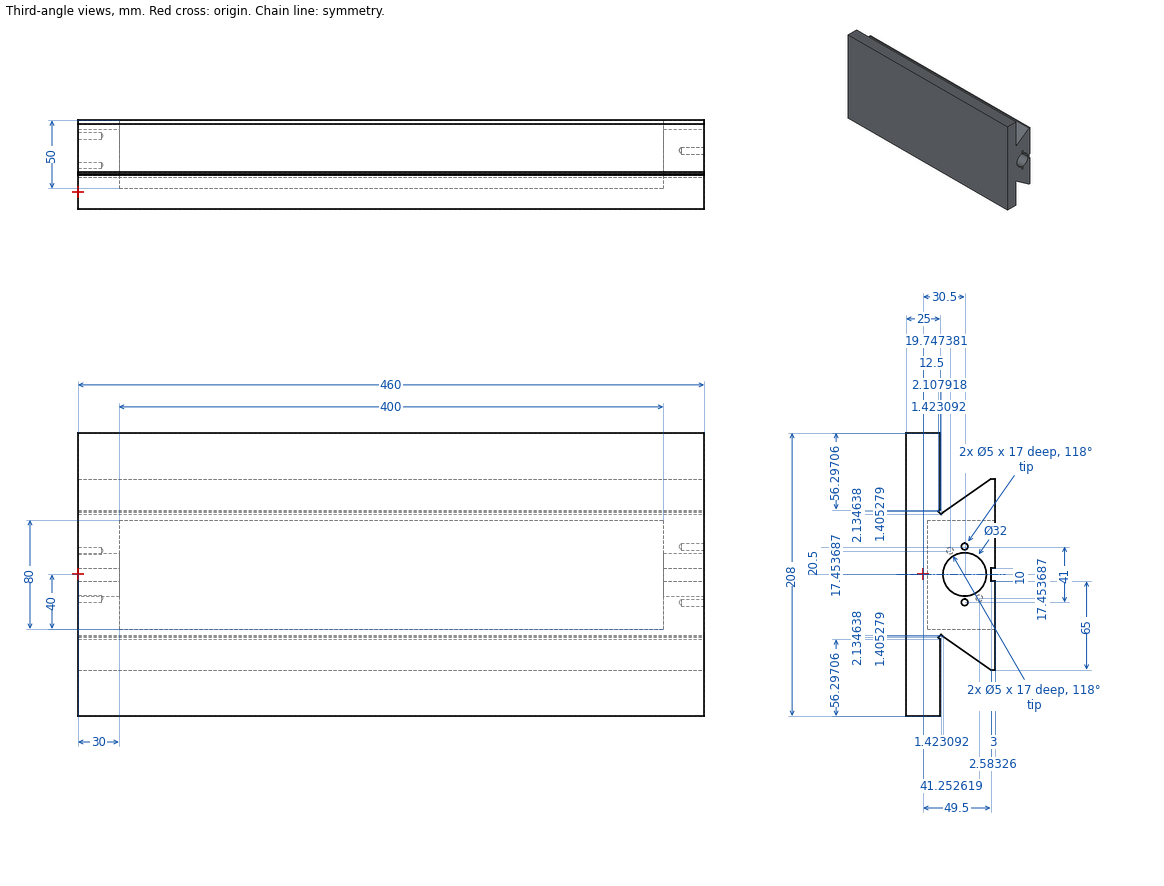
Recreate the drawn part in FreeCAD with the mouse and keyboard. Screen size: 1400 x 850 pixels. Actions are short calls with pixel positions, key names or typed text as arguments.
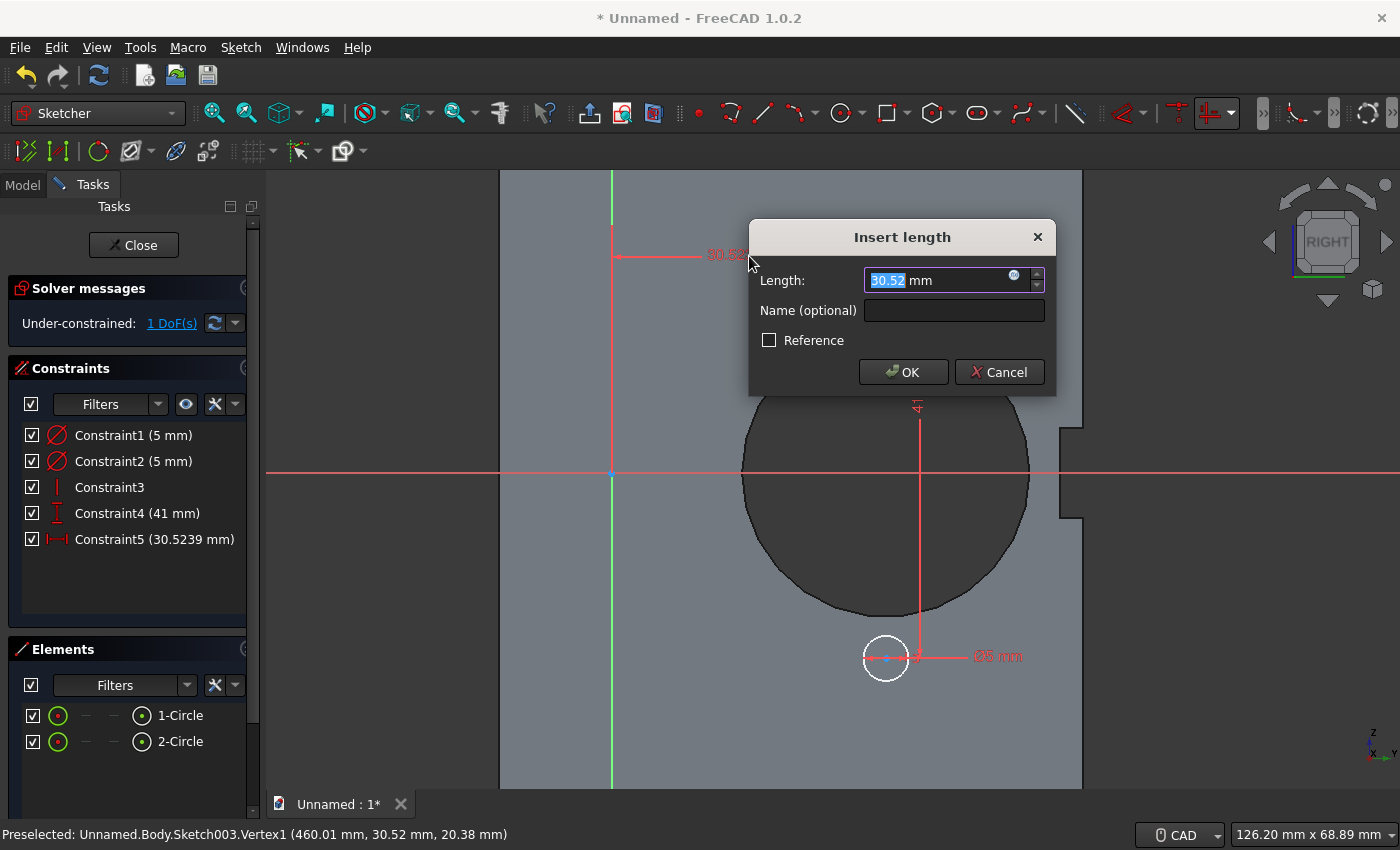
text(30.5)
key(Return)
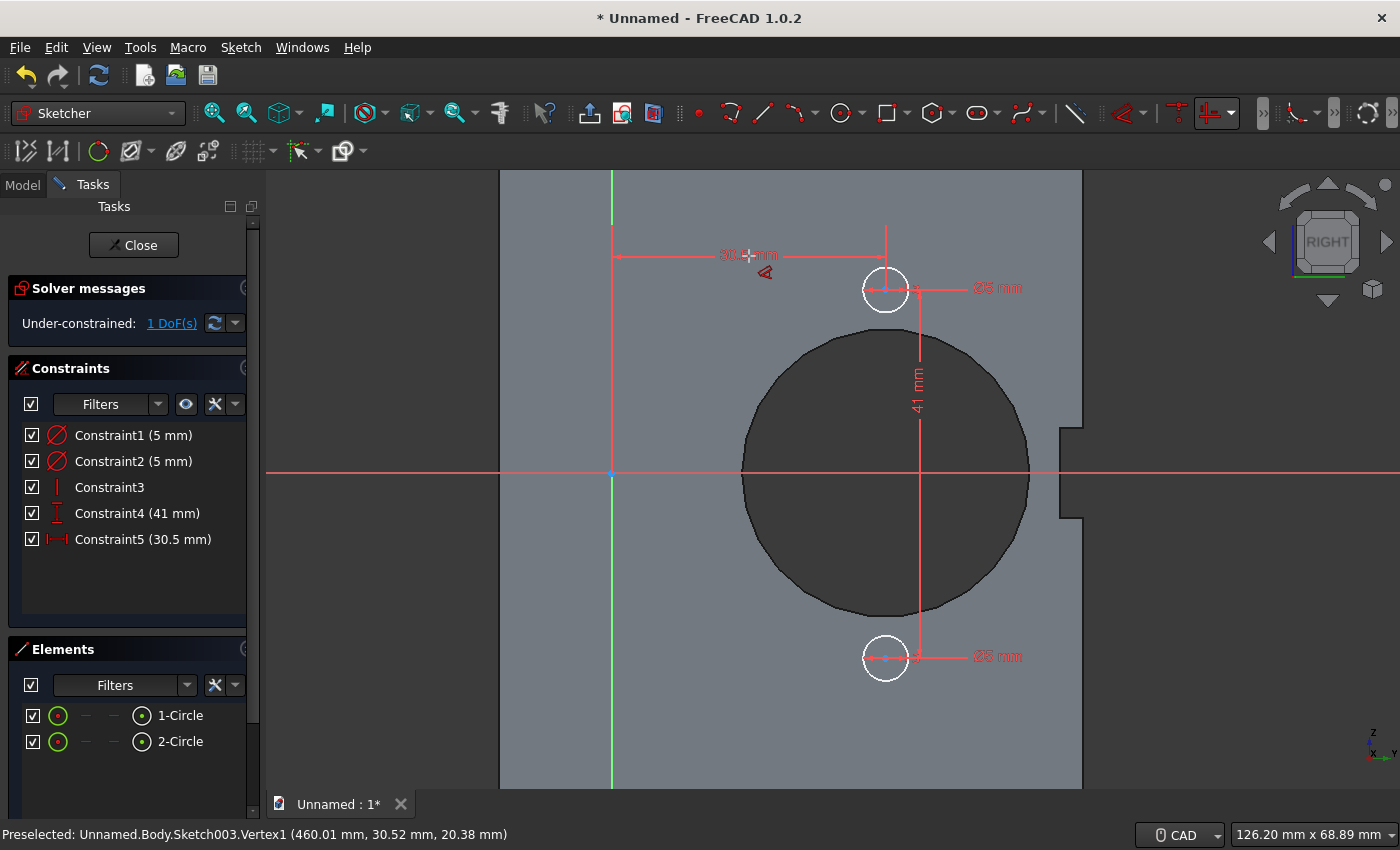
click(886, 290)
click(578, 382)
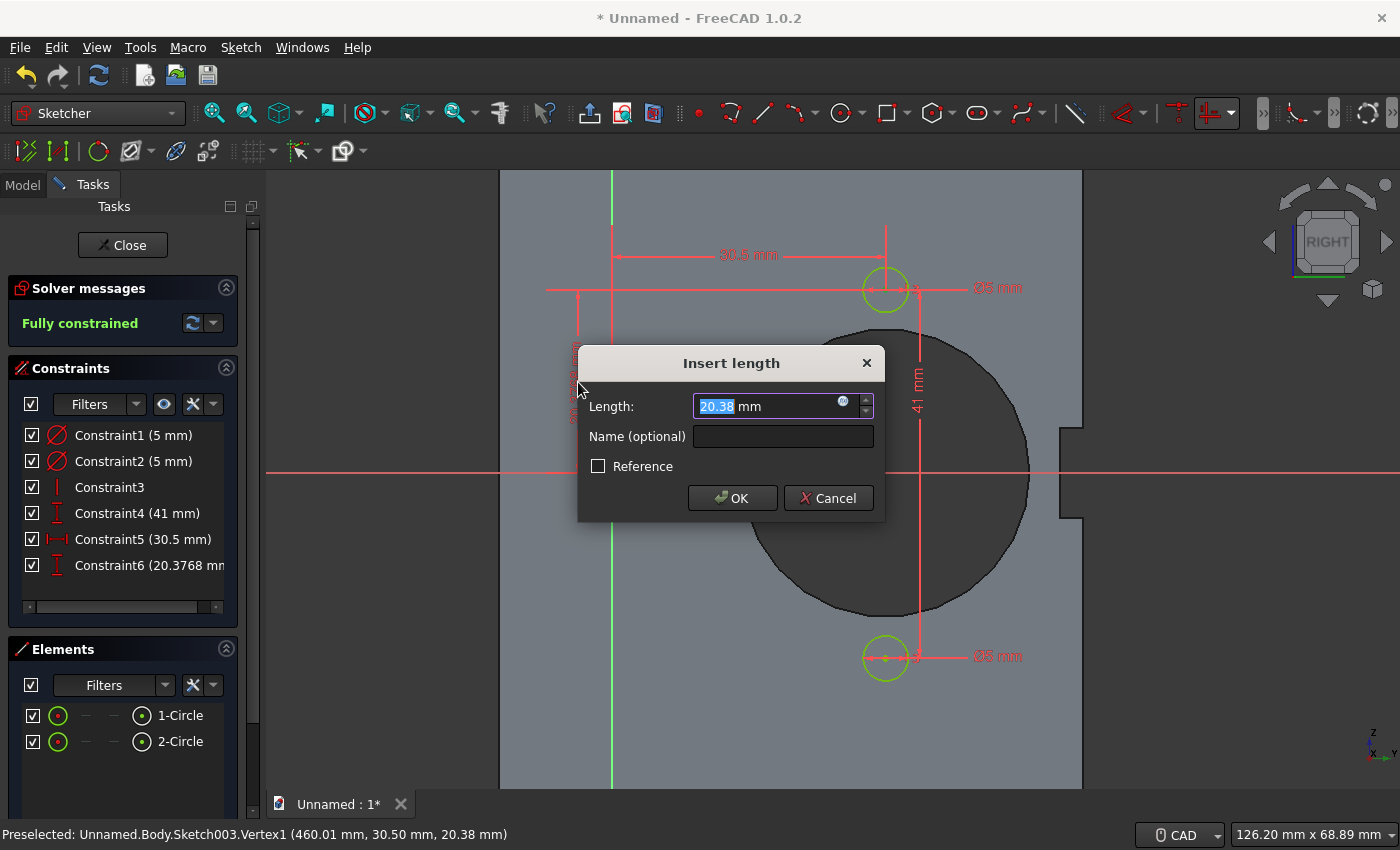
text(20.5)
key(Return)
key(Escape)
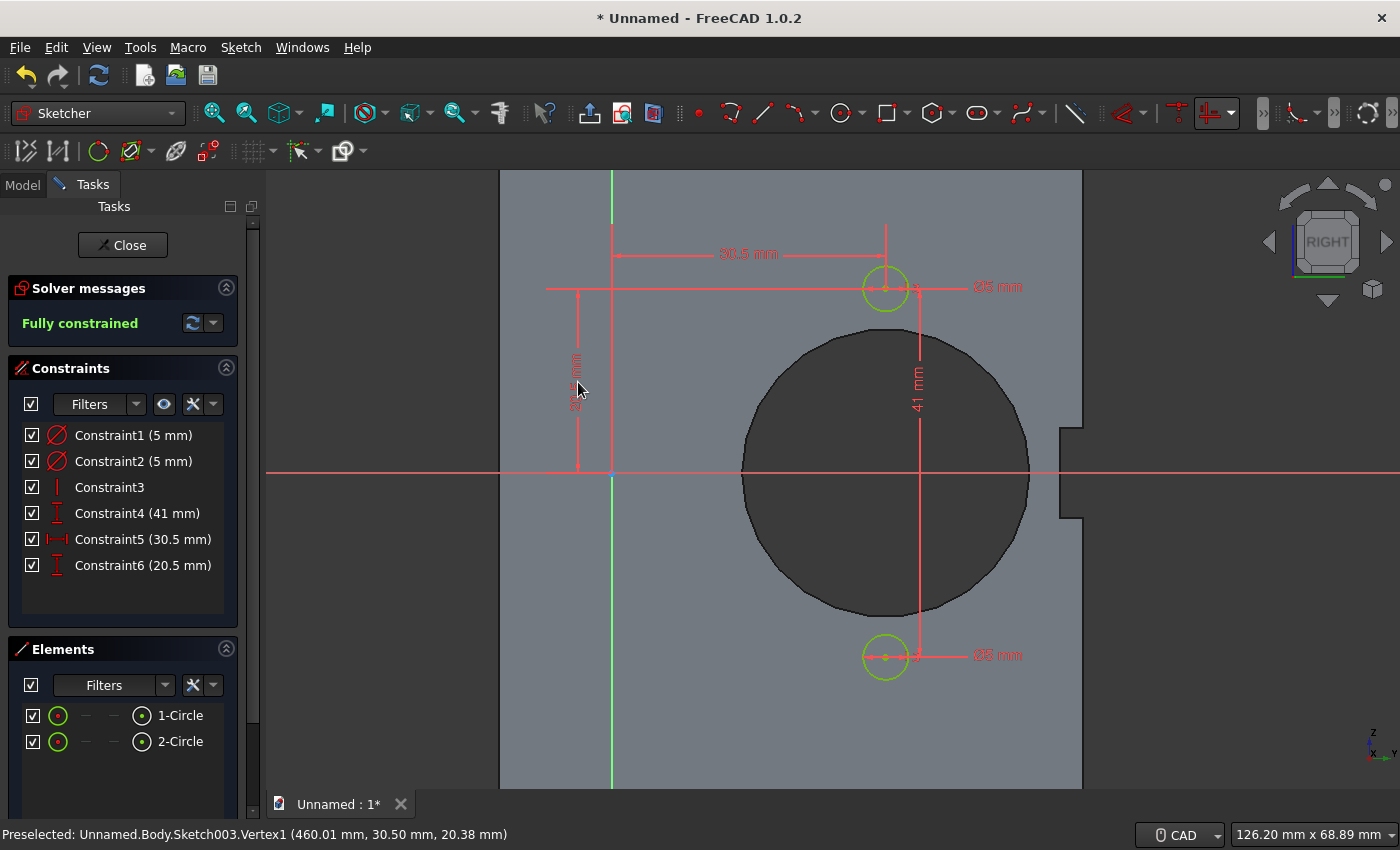
click(123, 245)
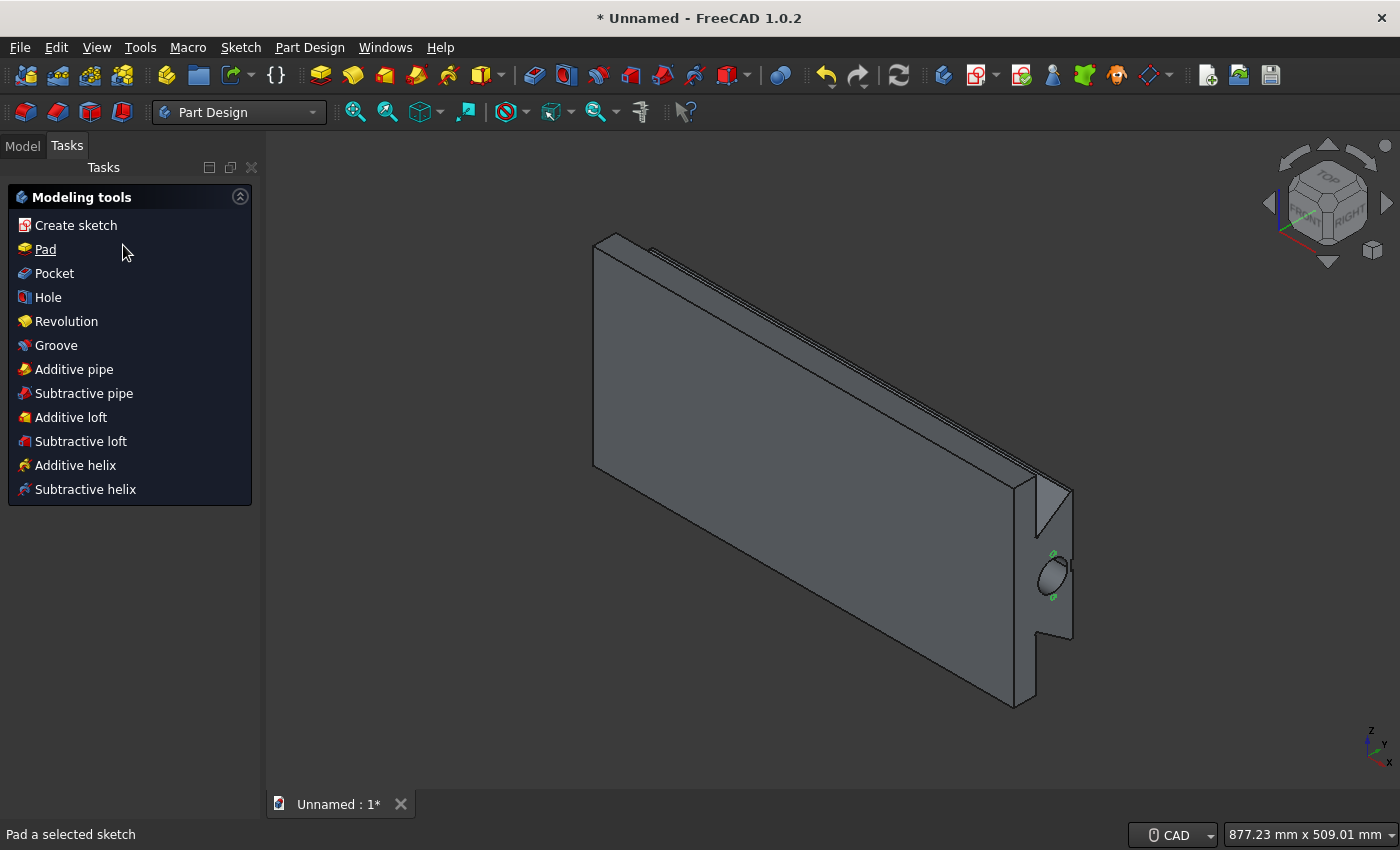
click(568, 76)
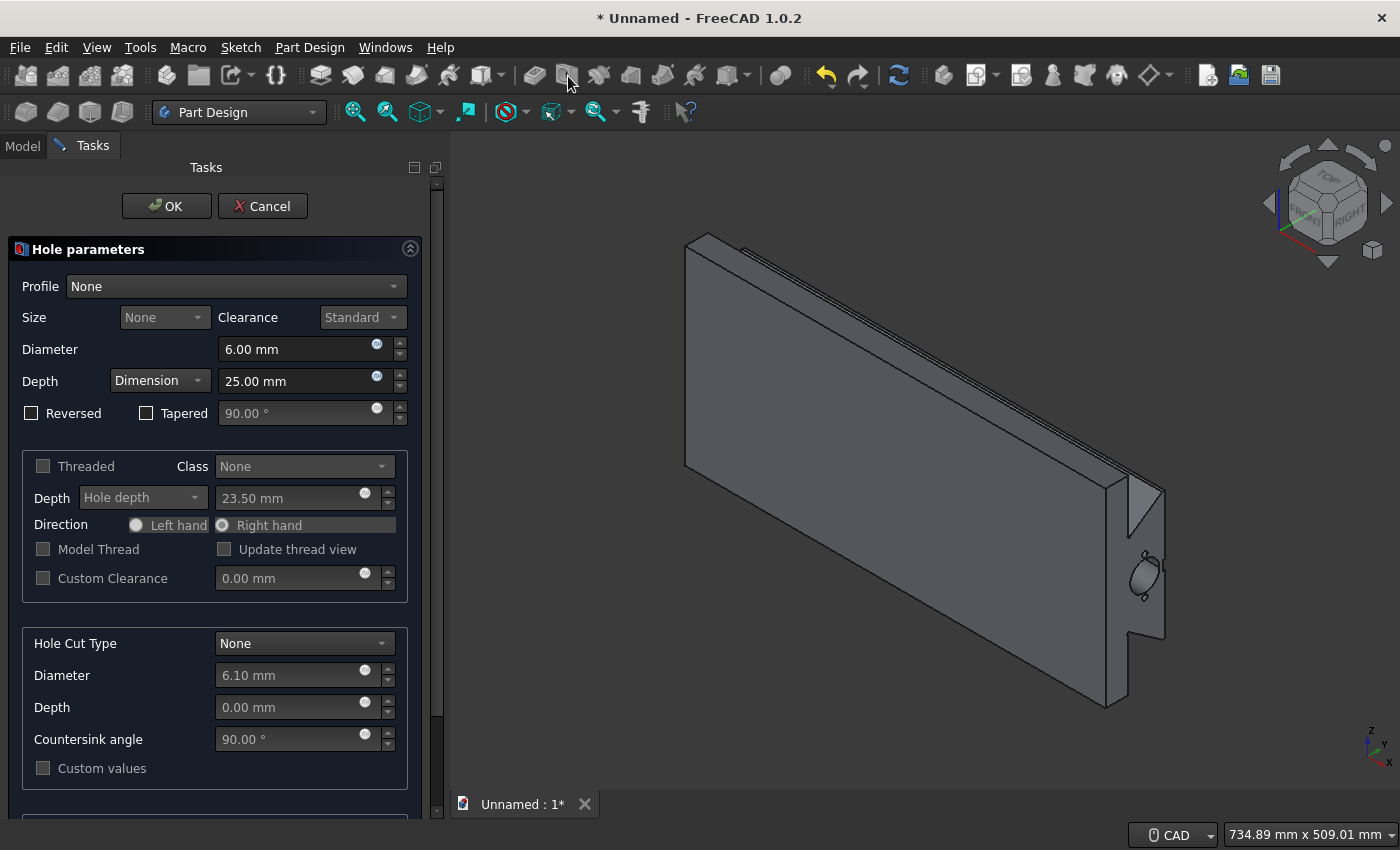
triple_click(305, 349)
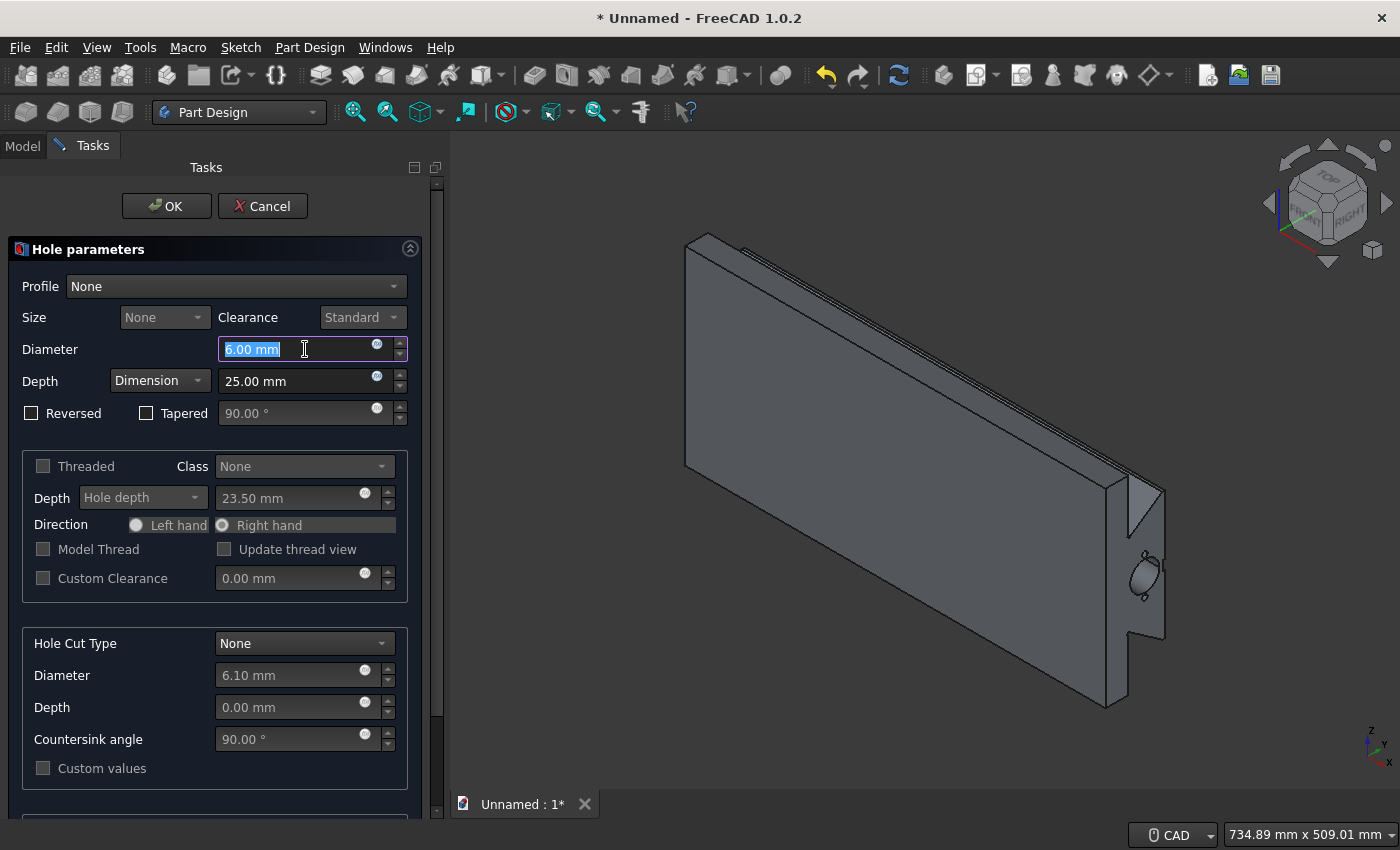
text(5)
key(Tab)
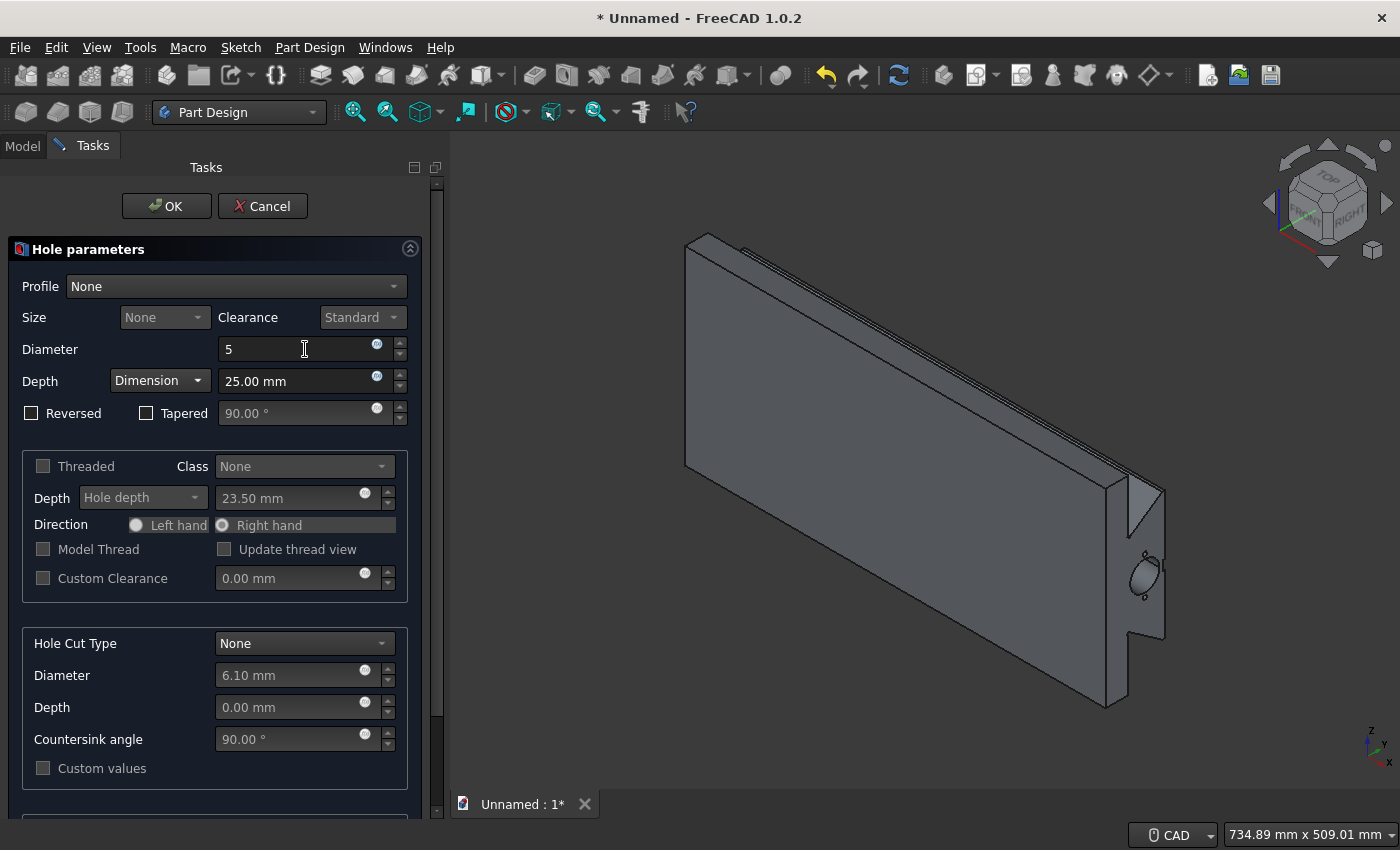
triple_click(305, 381)